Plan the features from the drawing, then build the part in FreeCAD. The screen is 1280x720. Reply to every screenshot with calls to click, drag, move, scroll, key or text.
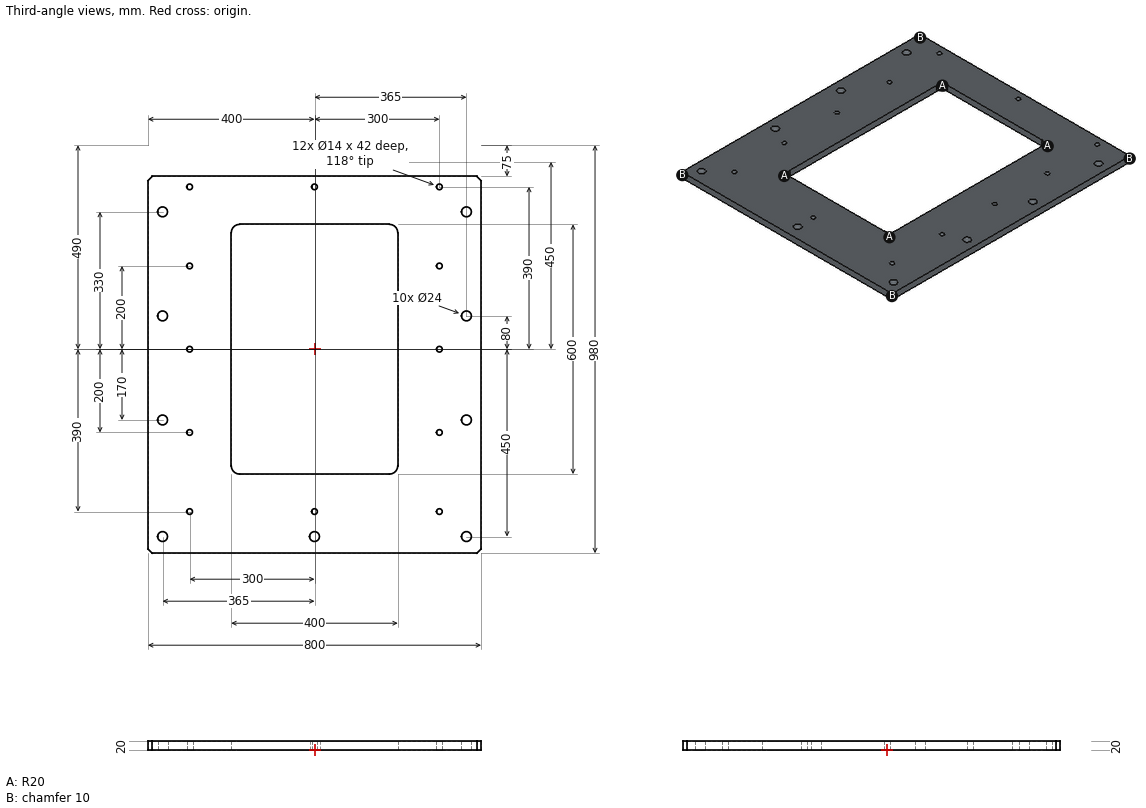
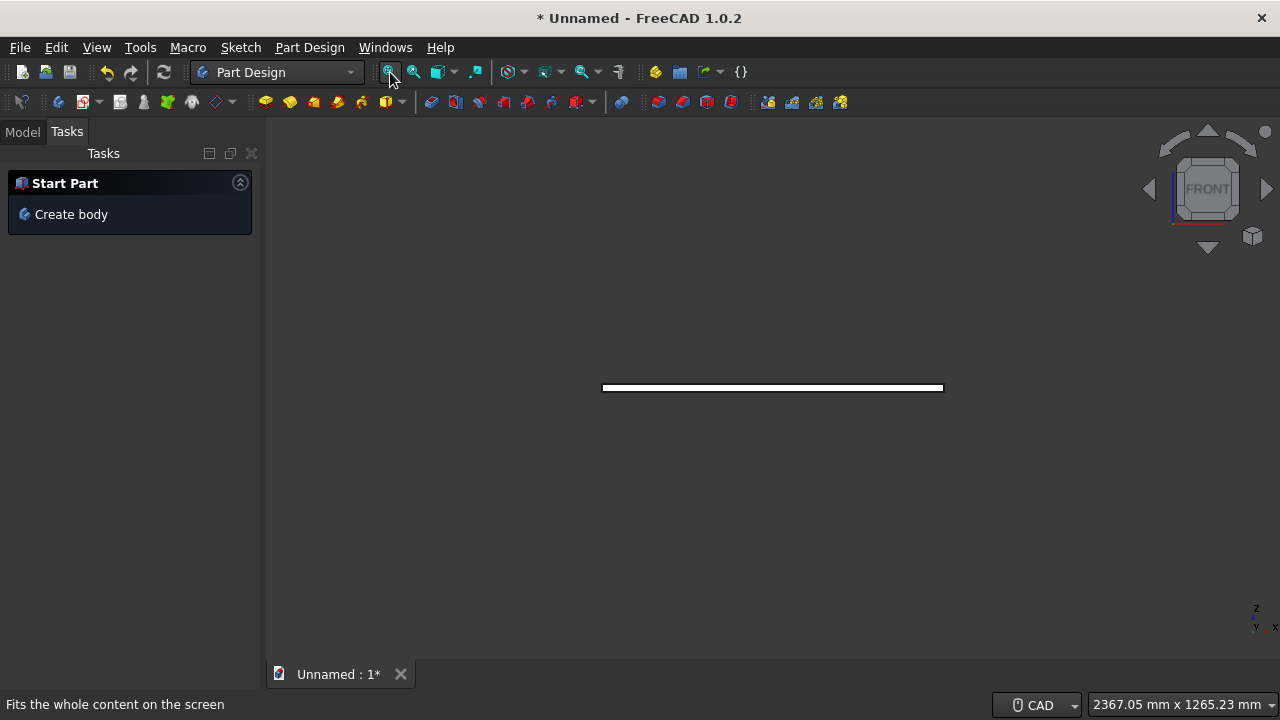
key(3)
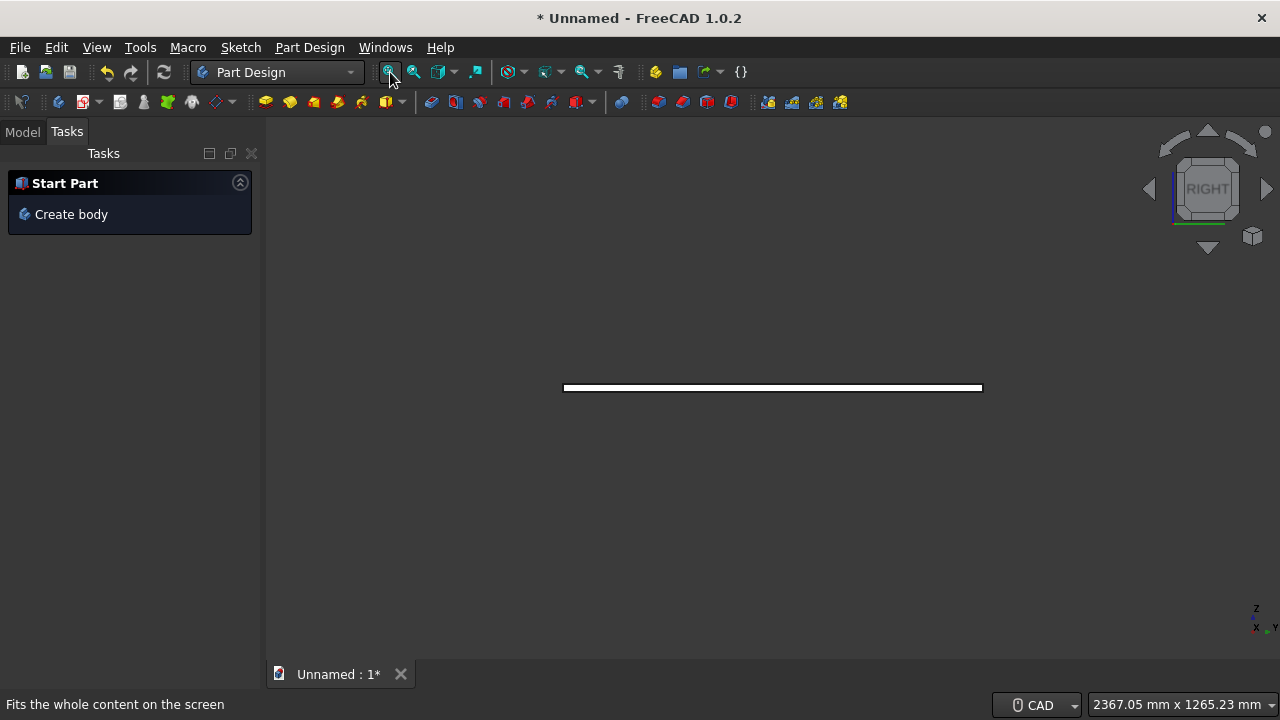
click(390, 72)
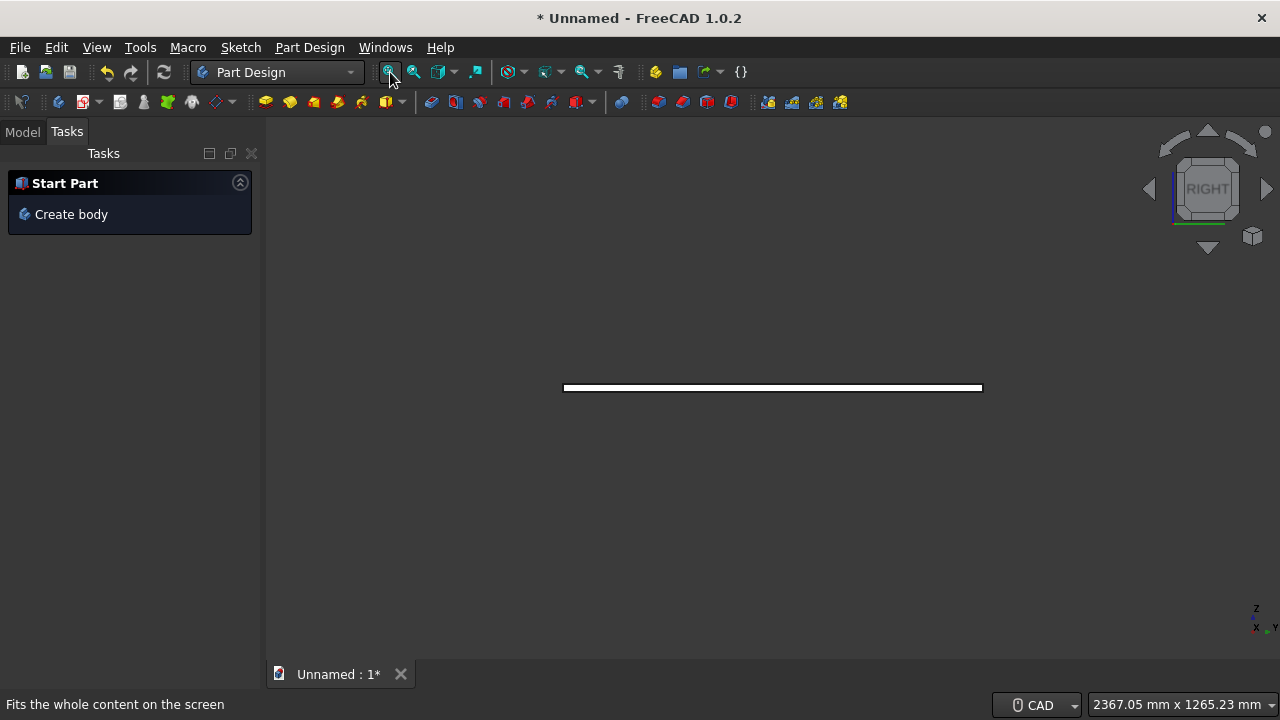
scroll(902, 387, up, 8)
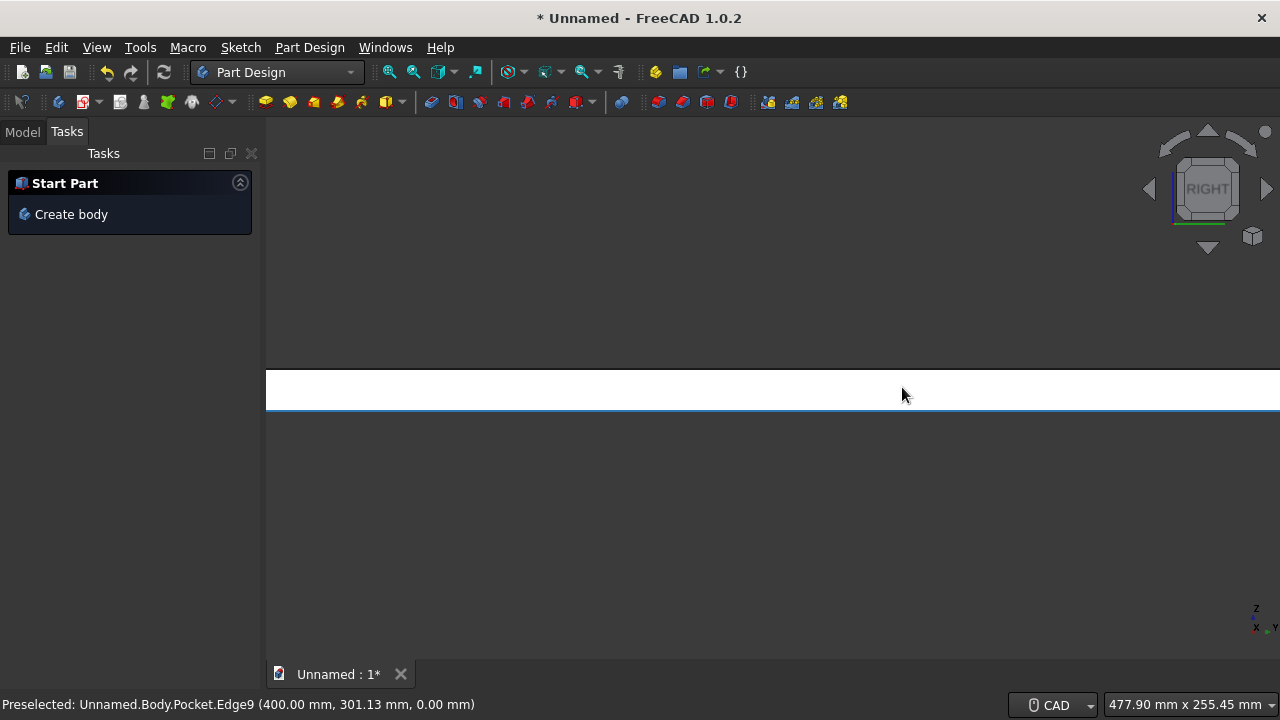
click(390, 72)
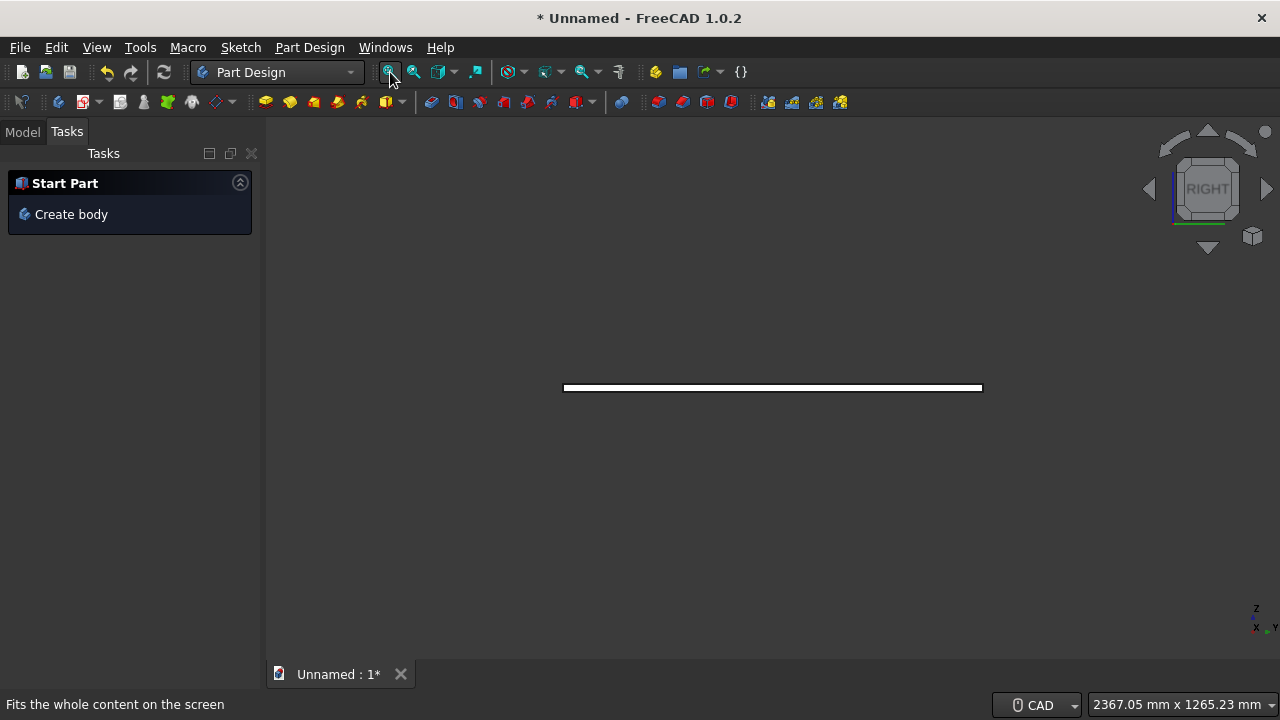
key(5)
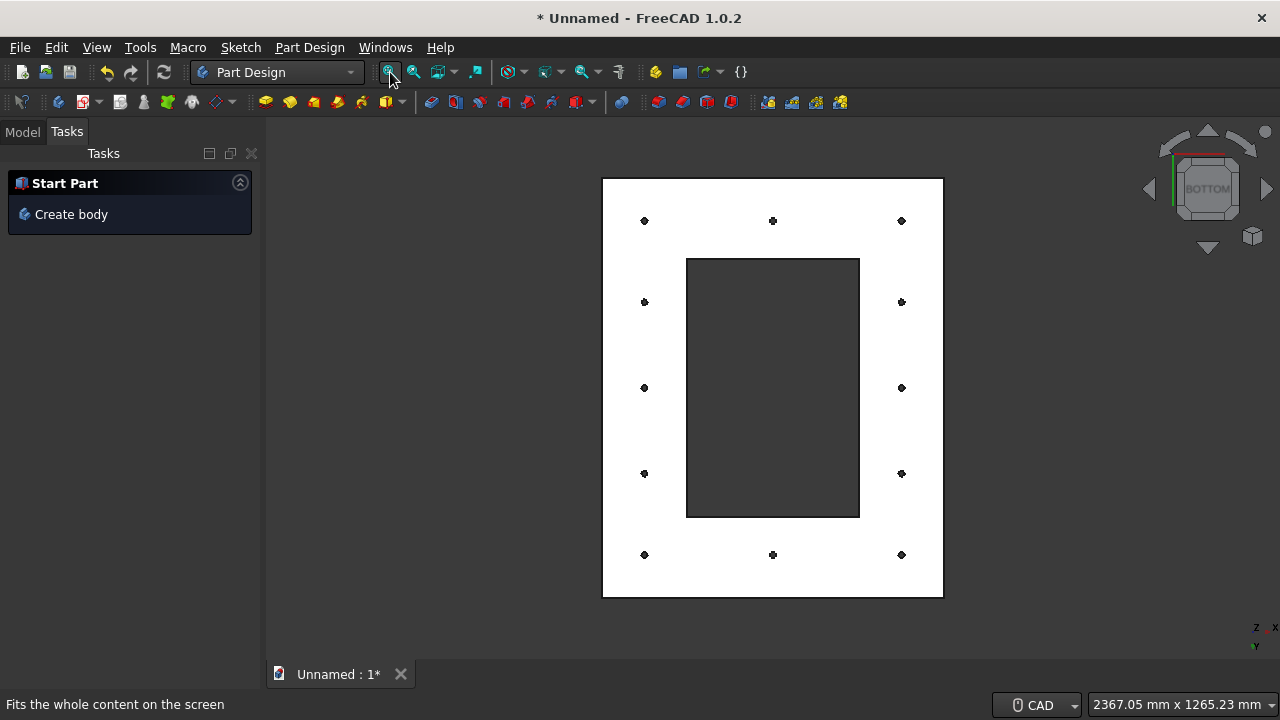
scroll(859, 516, up, 8)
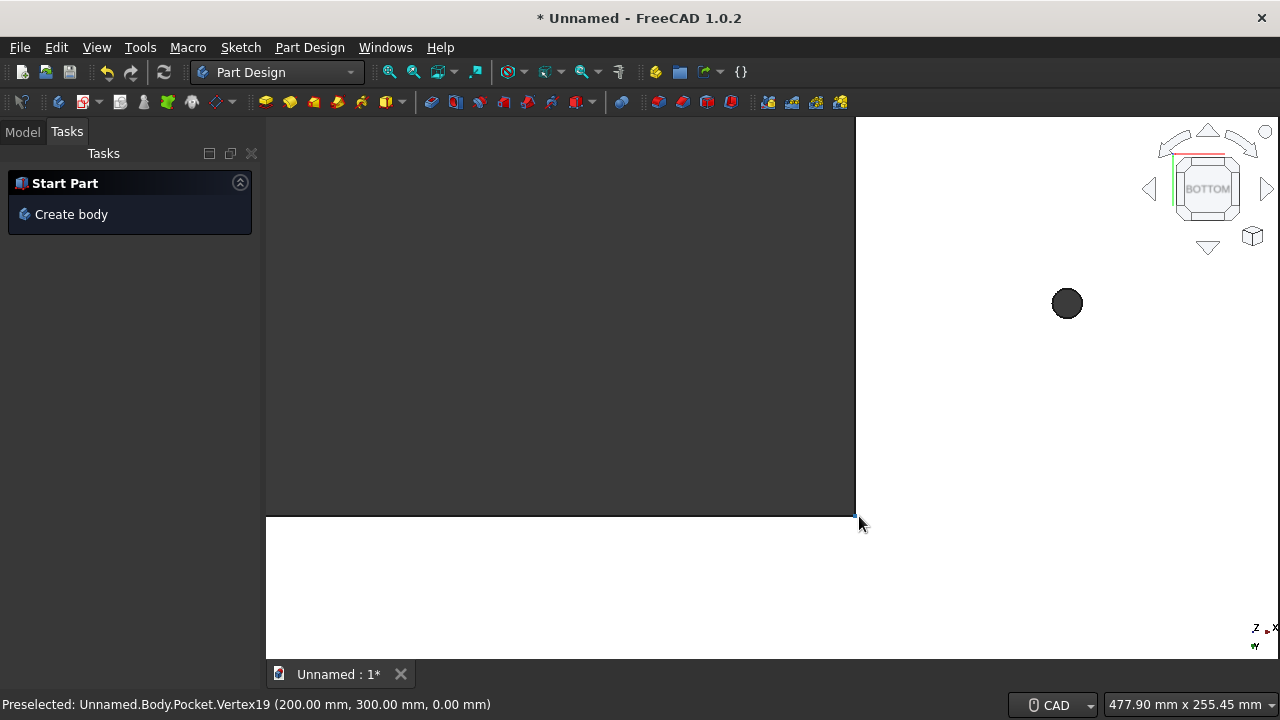
click(390, 72)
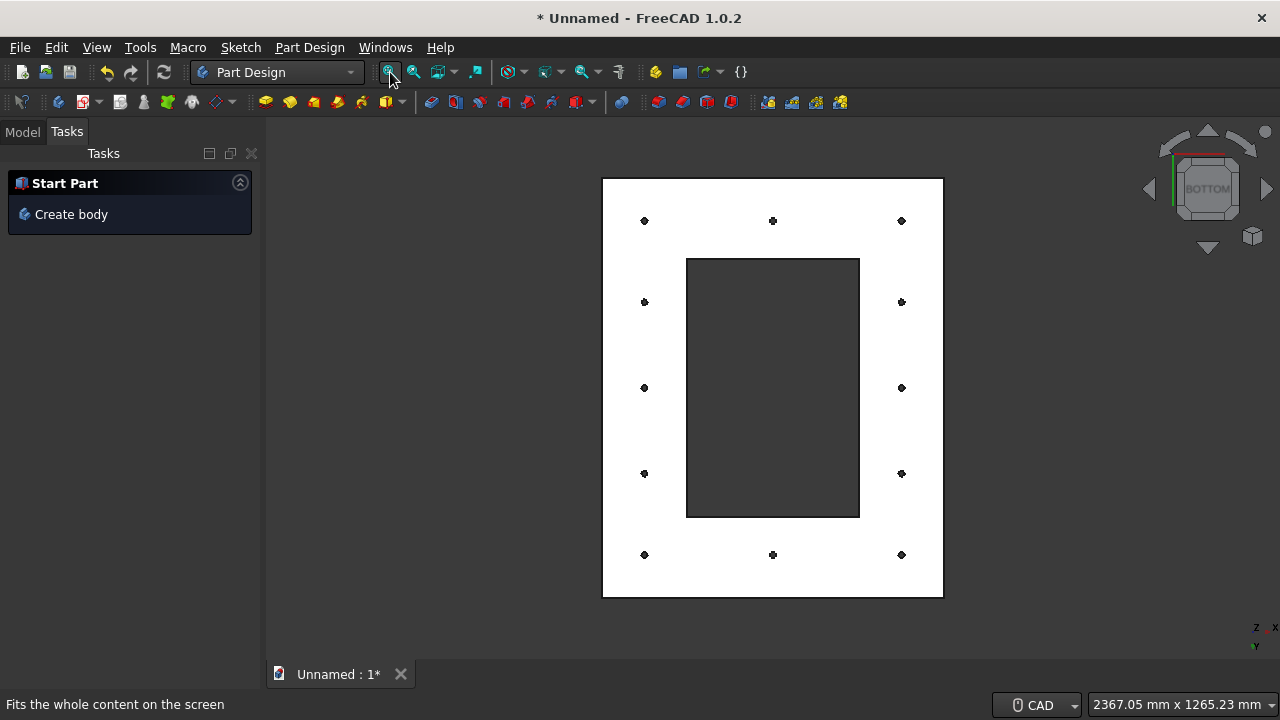
key(4)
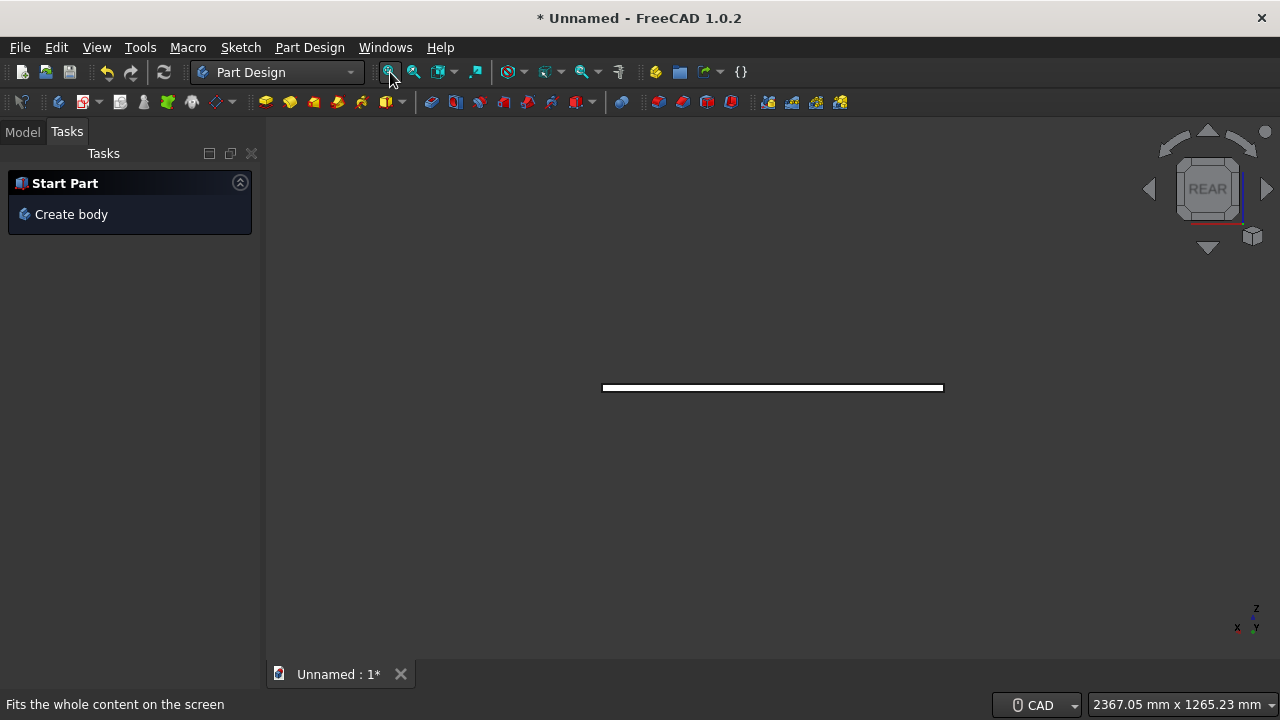
click(390, 72)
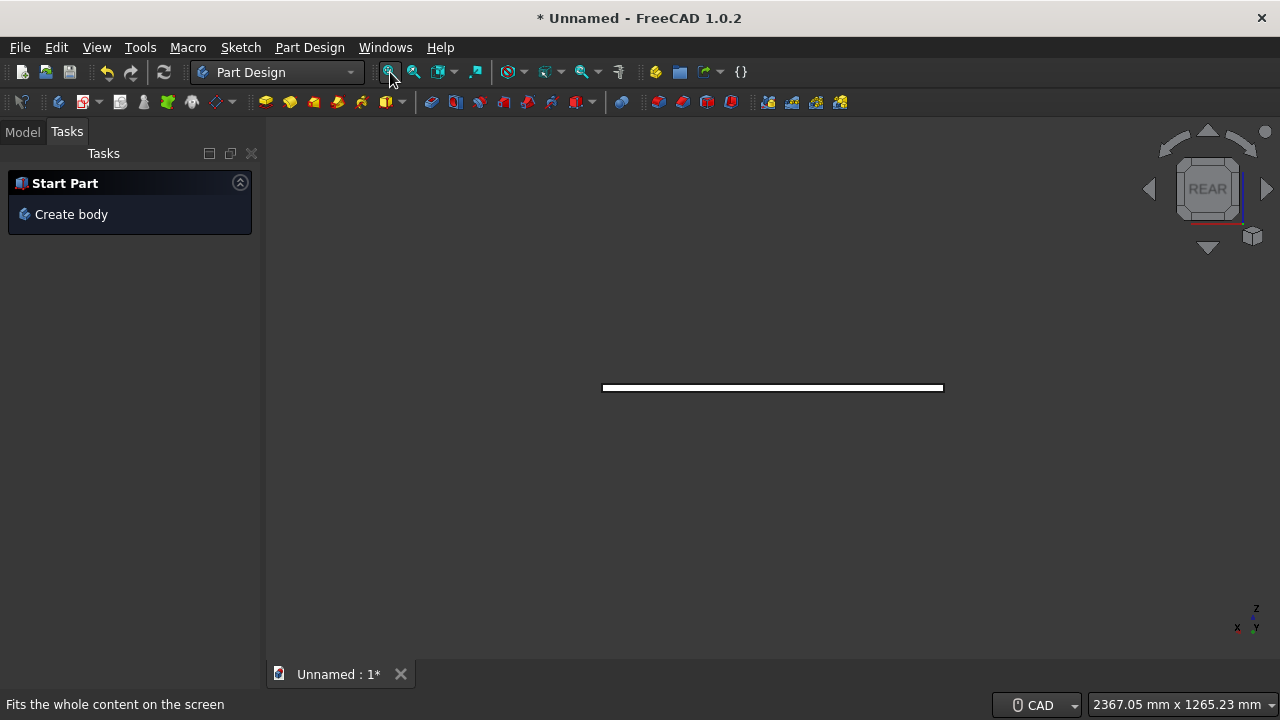
scroll(687, 387, up, 8)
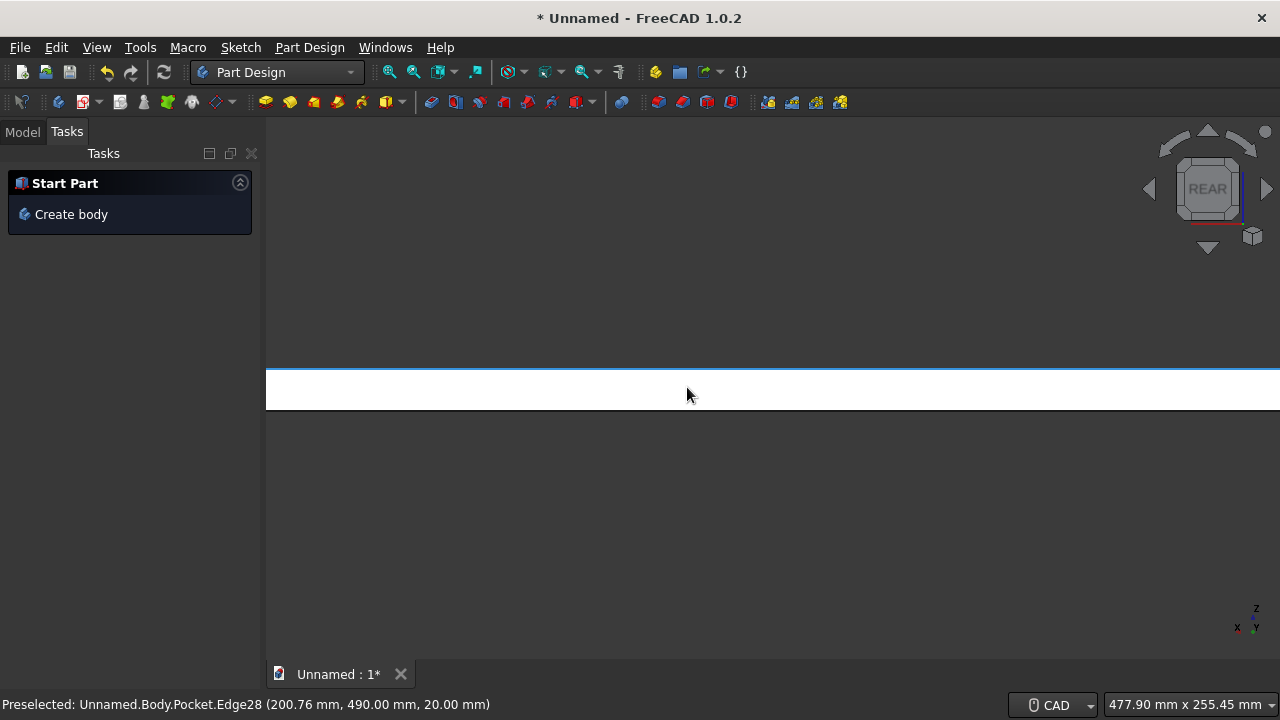
click(390, 72)